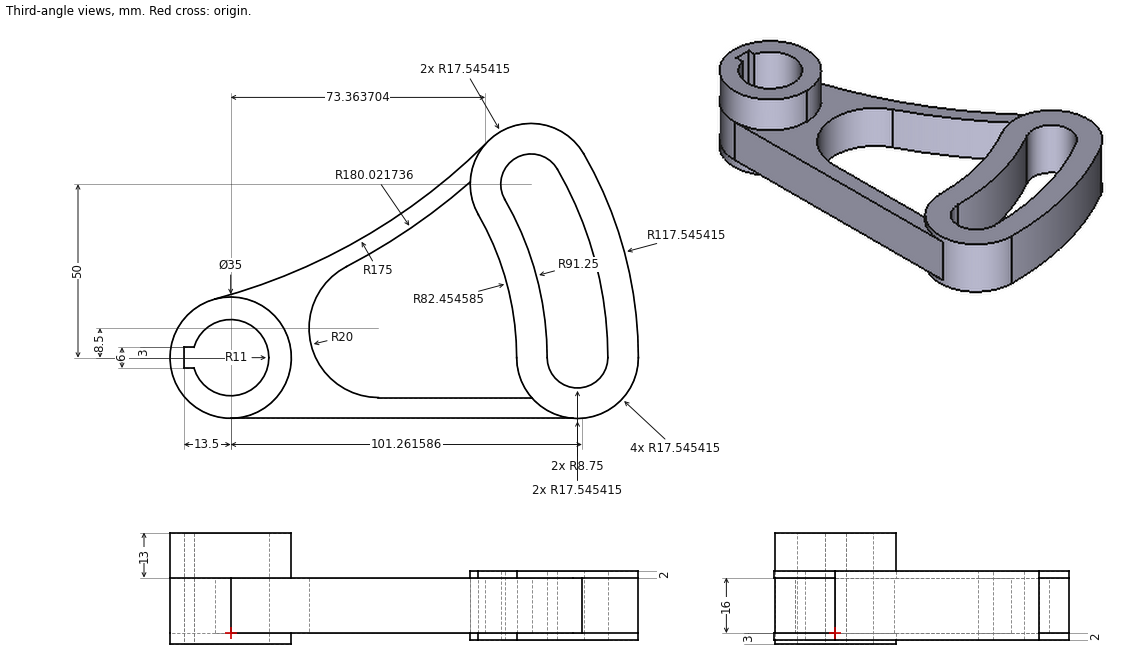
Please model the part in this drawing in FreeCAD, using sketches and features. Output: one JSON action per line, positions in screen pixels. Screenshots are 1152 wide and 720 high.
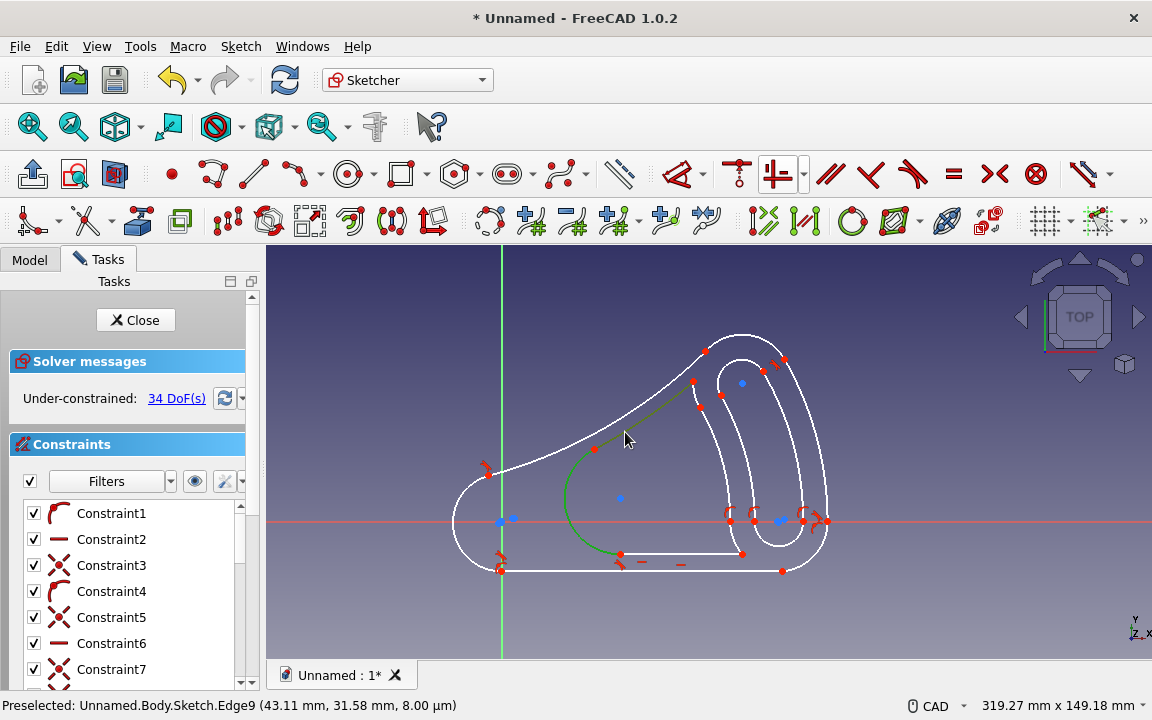
{"action": "left_click", "coordinate": [913, 174]}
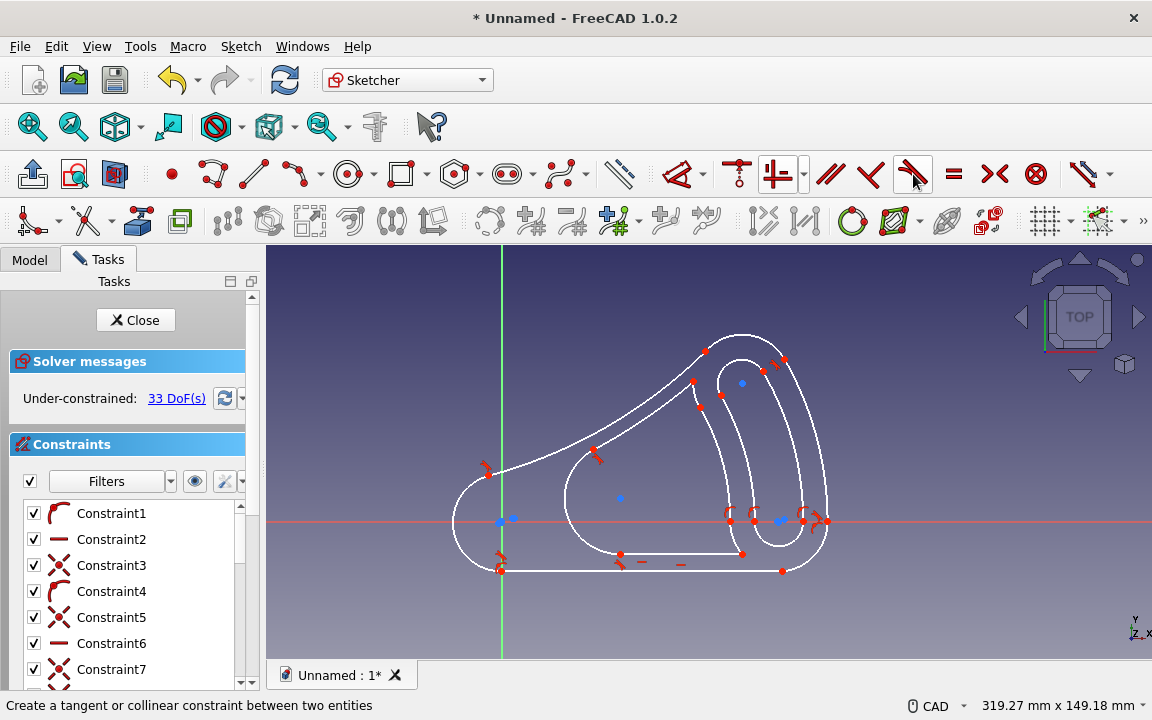
{"action": "left_click", "coordinate": [695, 395]}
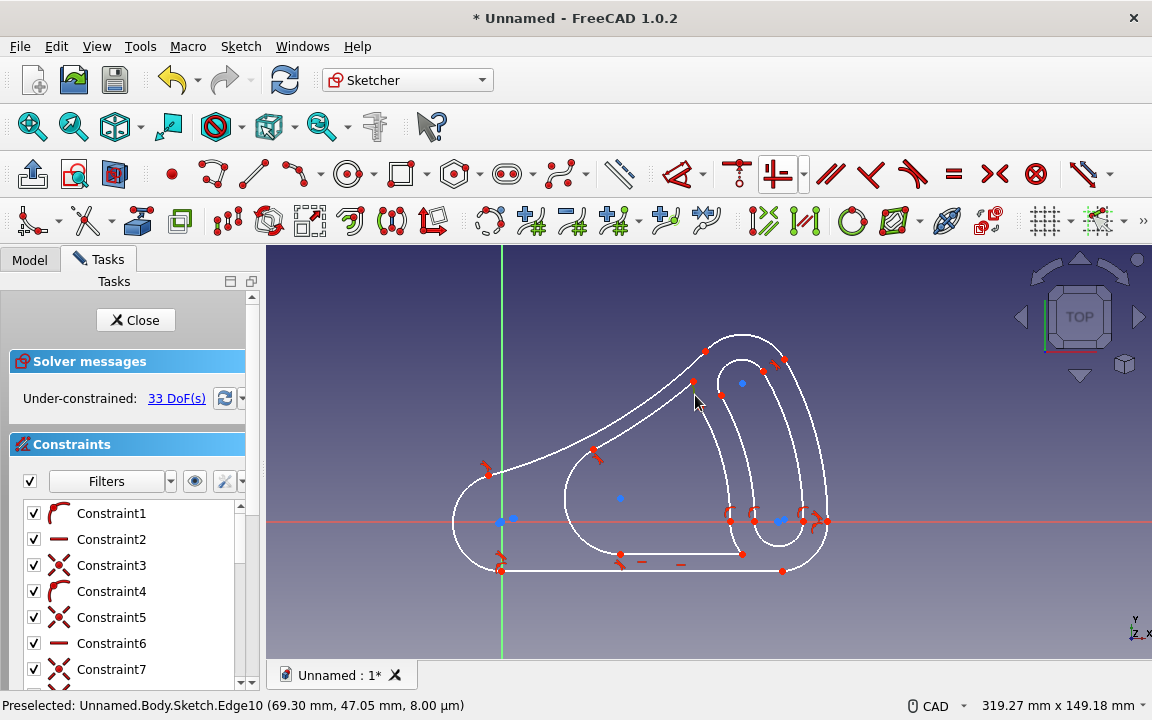
{"action": "left_click", "coordinate": [728, 486]}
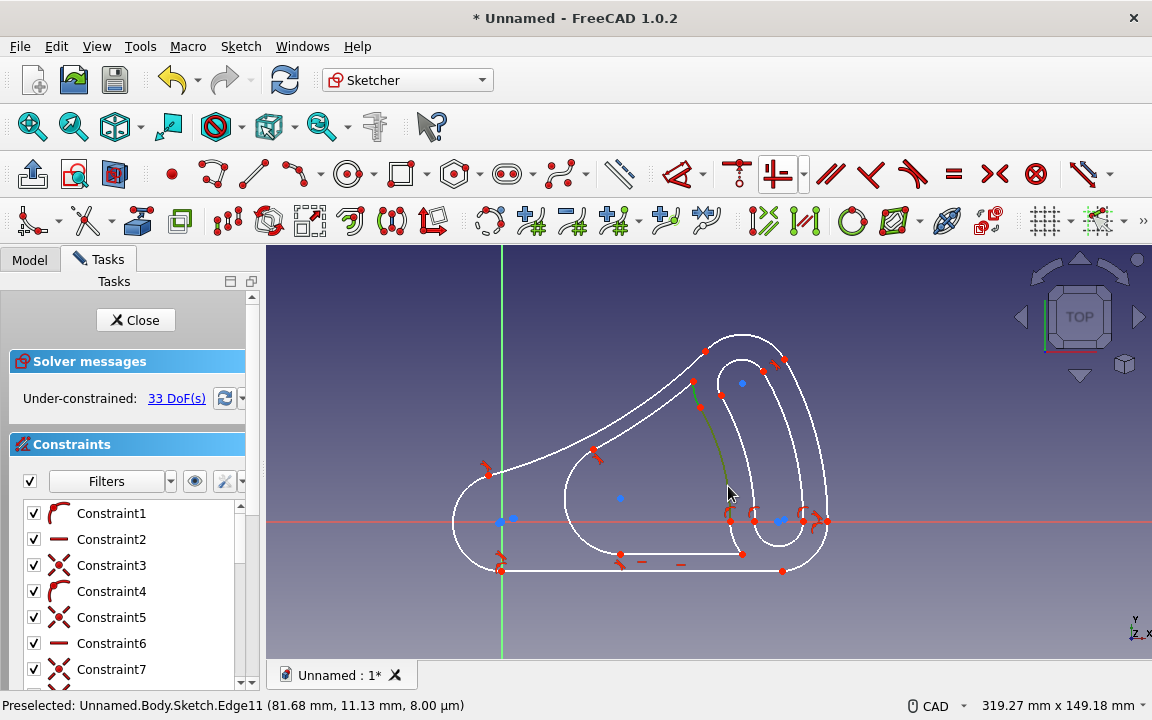
{"action": "left_click", "coordinate": [913, 174]}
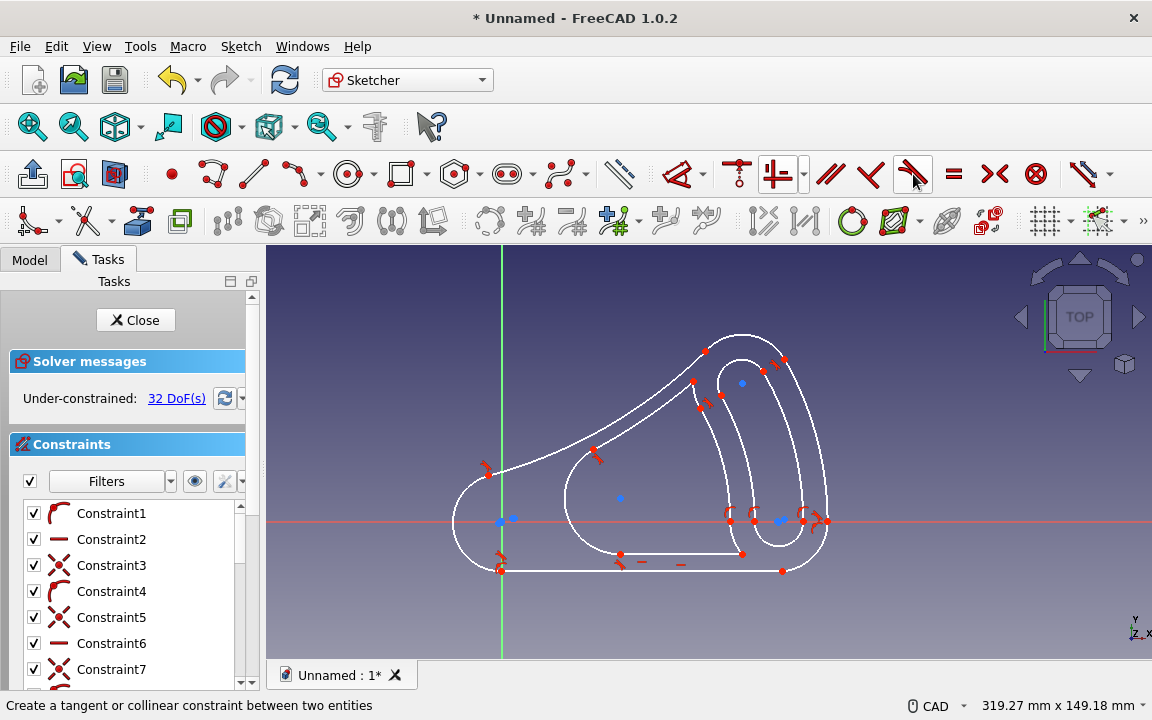
{"action": "left_click", "coordinate": [728, 486]}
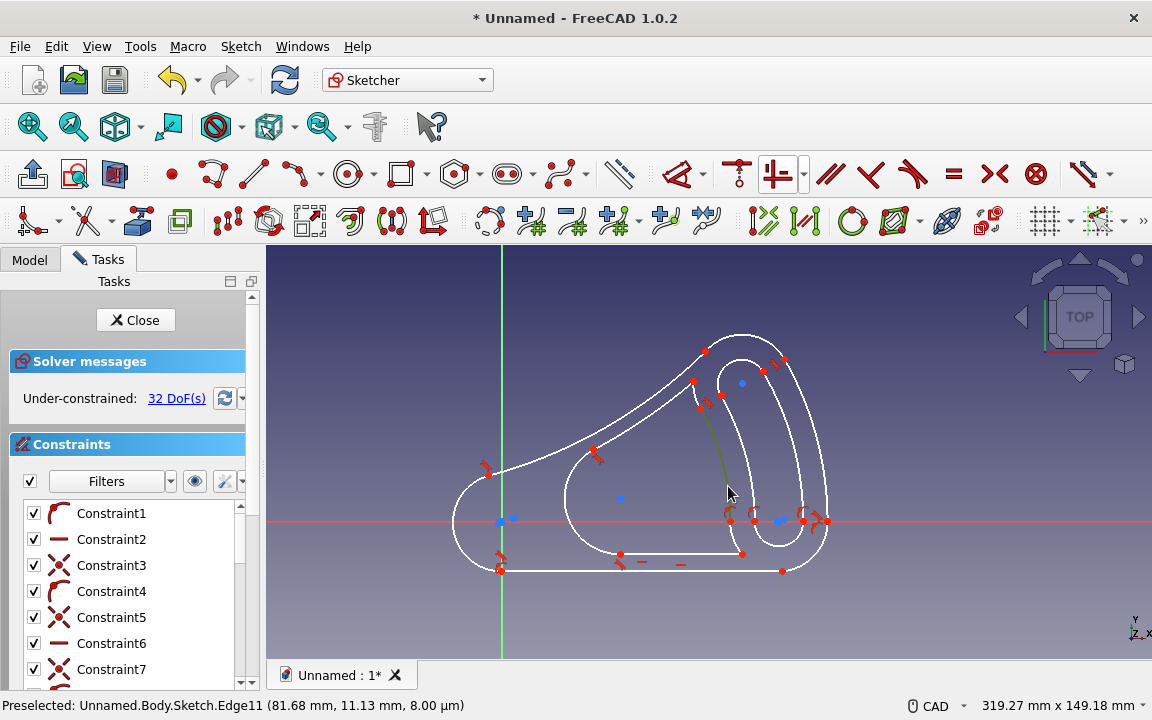
{"action": "scroll", "coordinate": [731, 532], "scroll_direction": "up", "scroll_amount": 2}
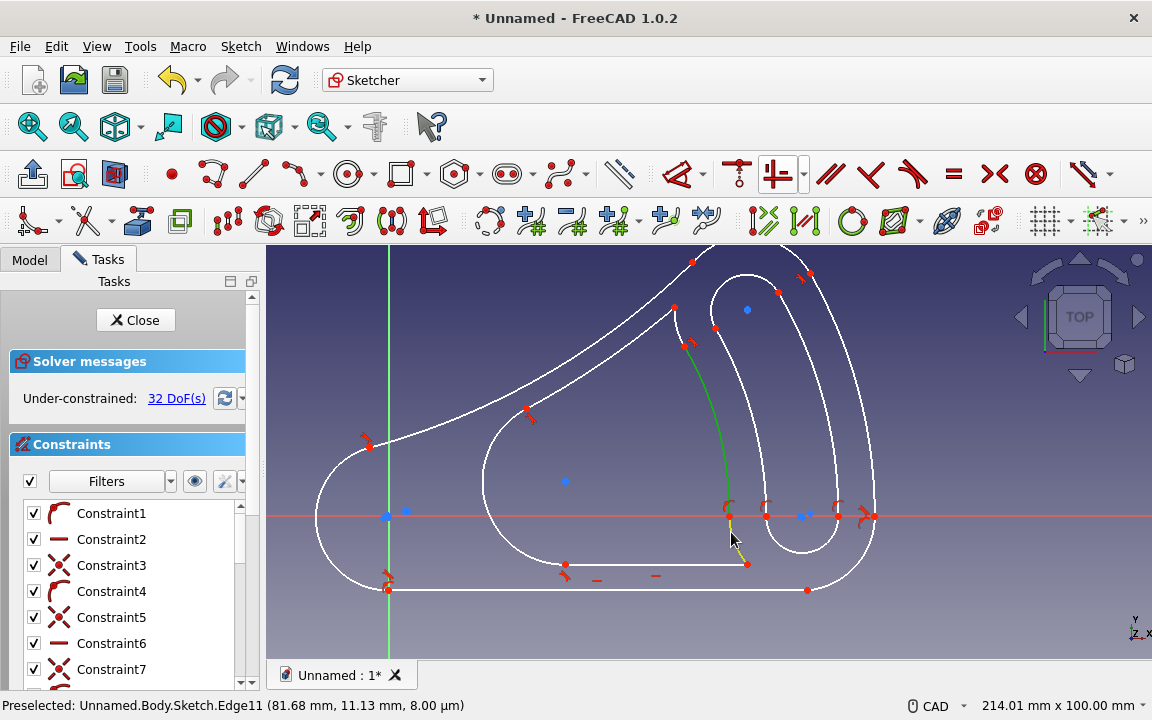
{"action": "left_click", "coordinate": [731, 532]}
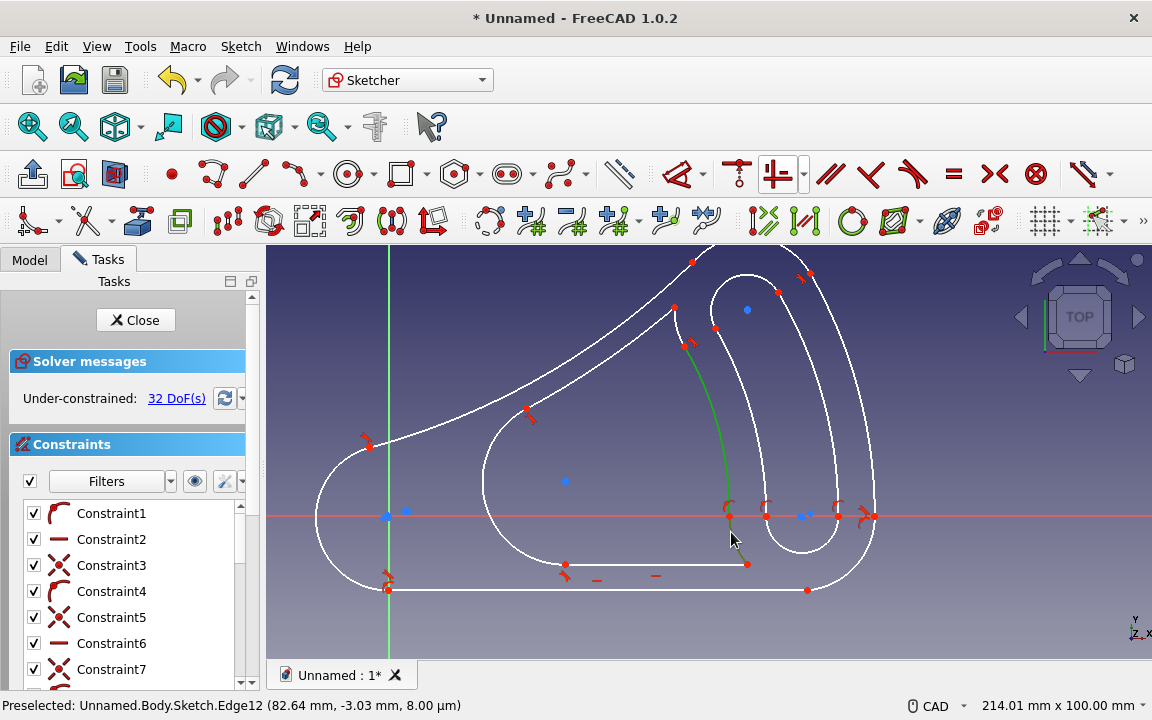
{"action": "left_click", "coordinate": [913, 174]}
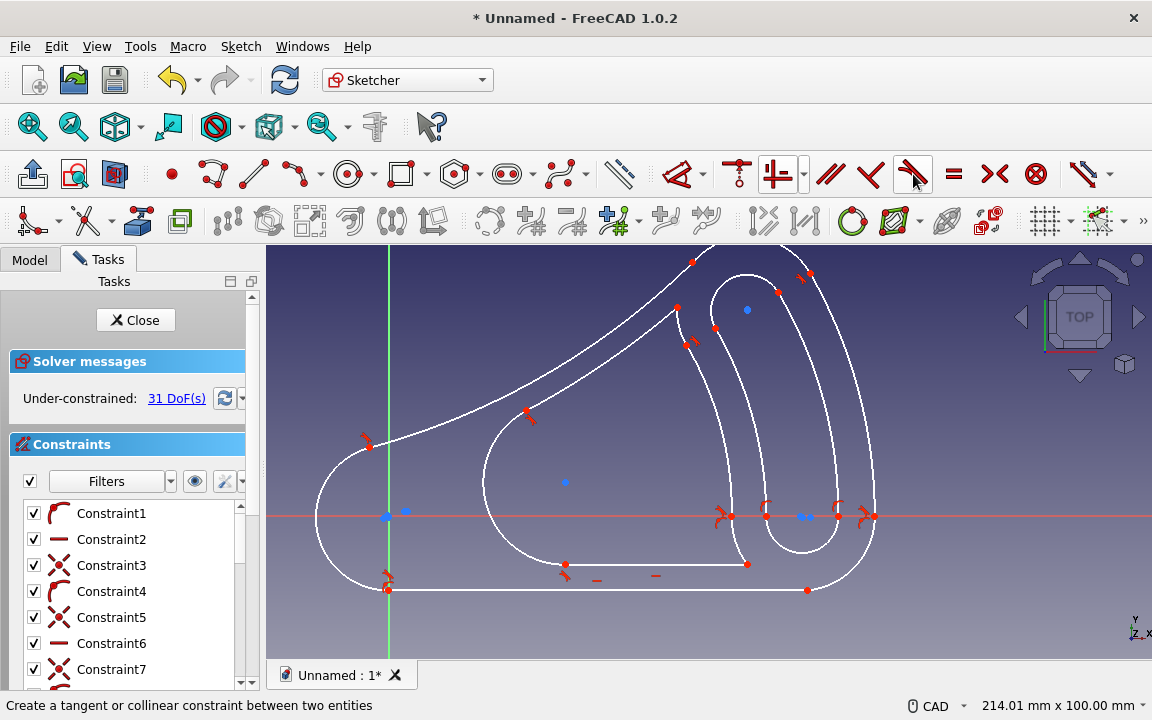
{"action": "left_click", "coordinate": [751, 275]}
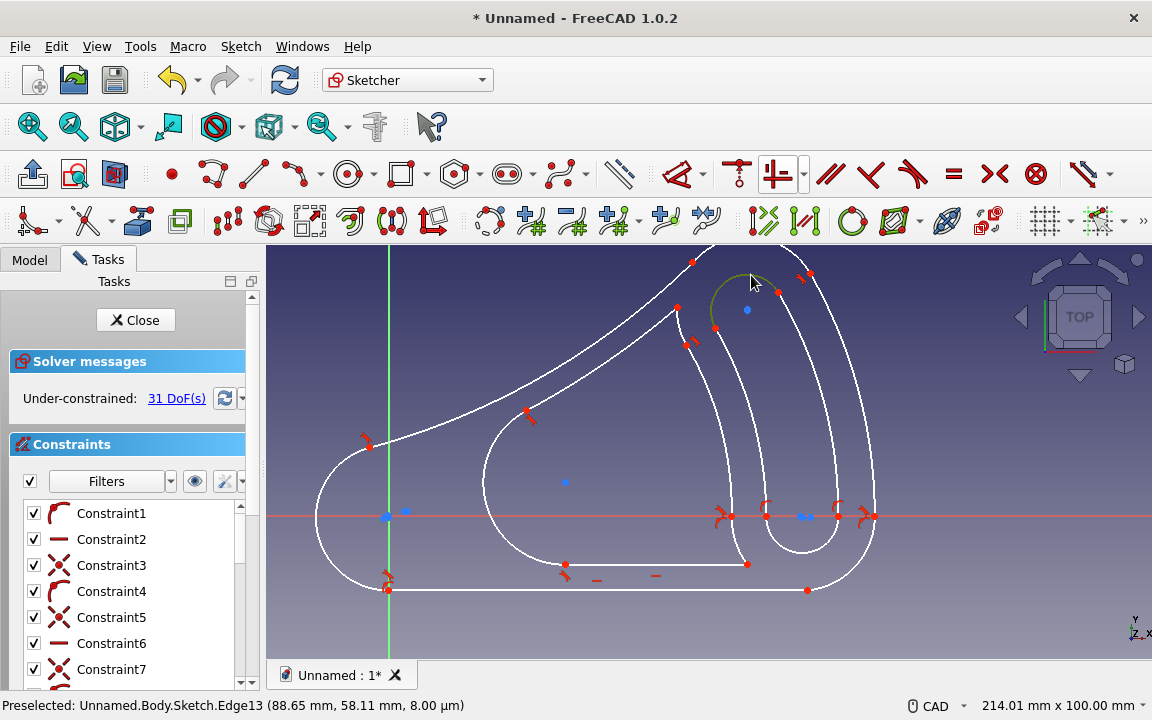
{"action": "left_click", "coordinate": [833, 446]}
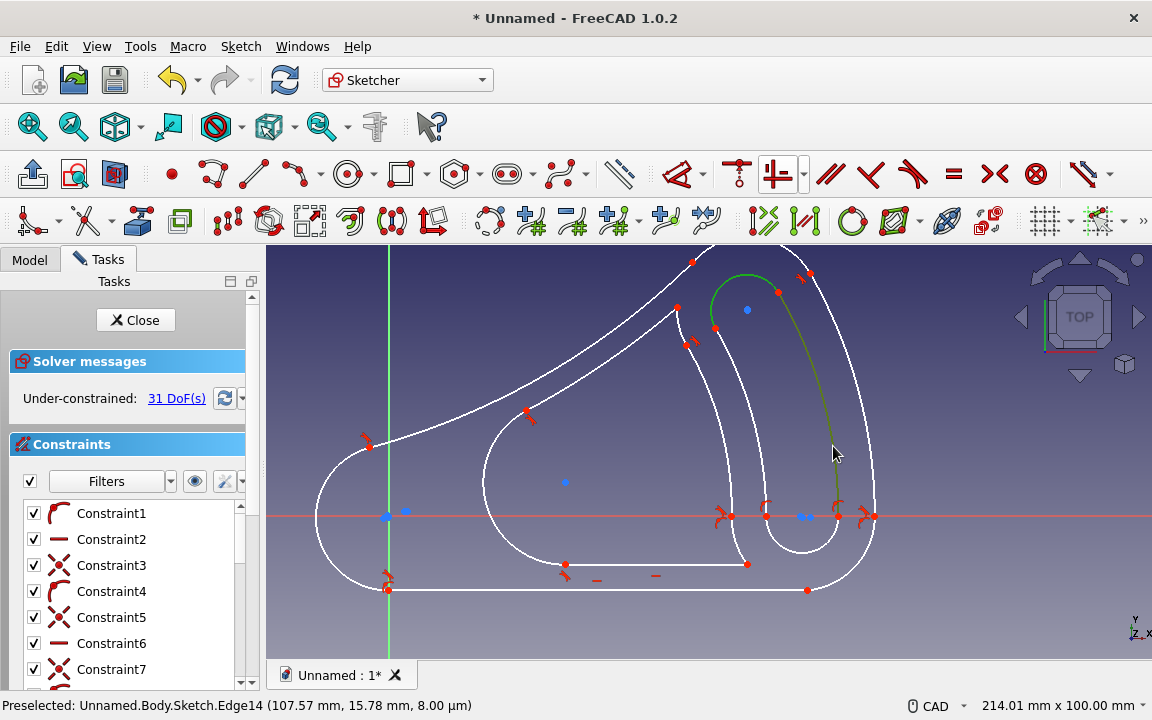
{"action": "left_click", "coordinate": [913, 174]}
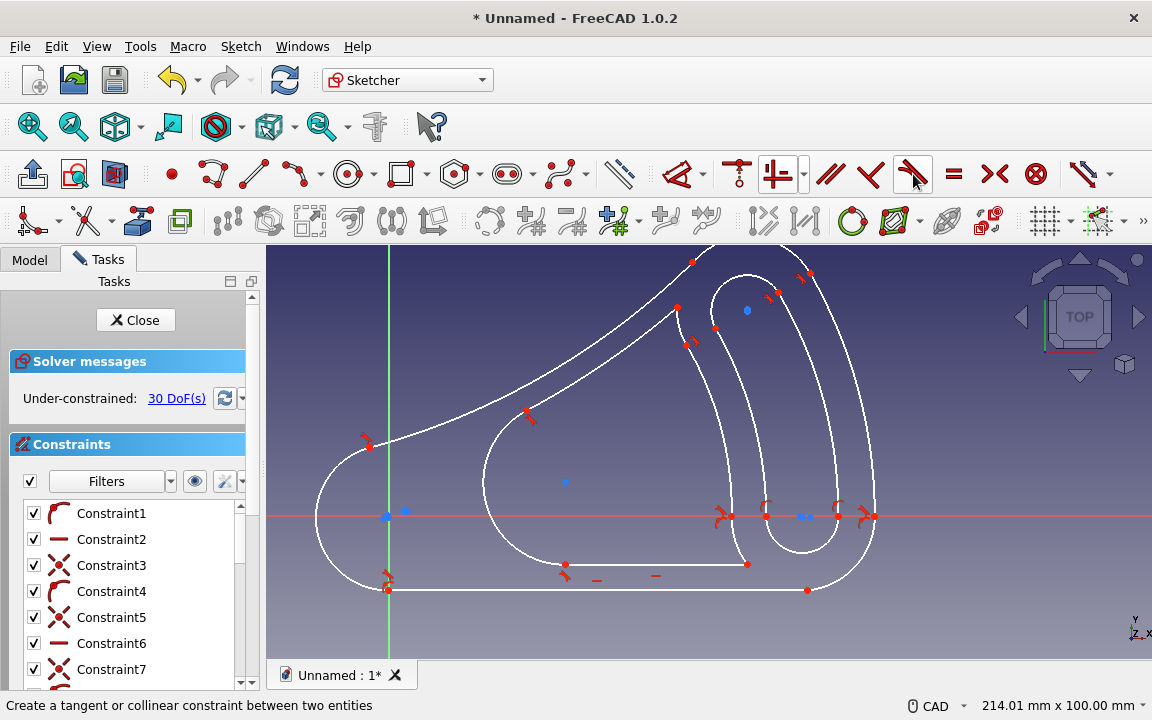
{"action": "left_click", "coordinate": [751, 275]}